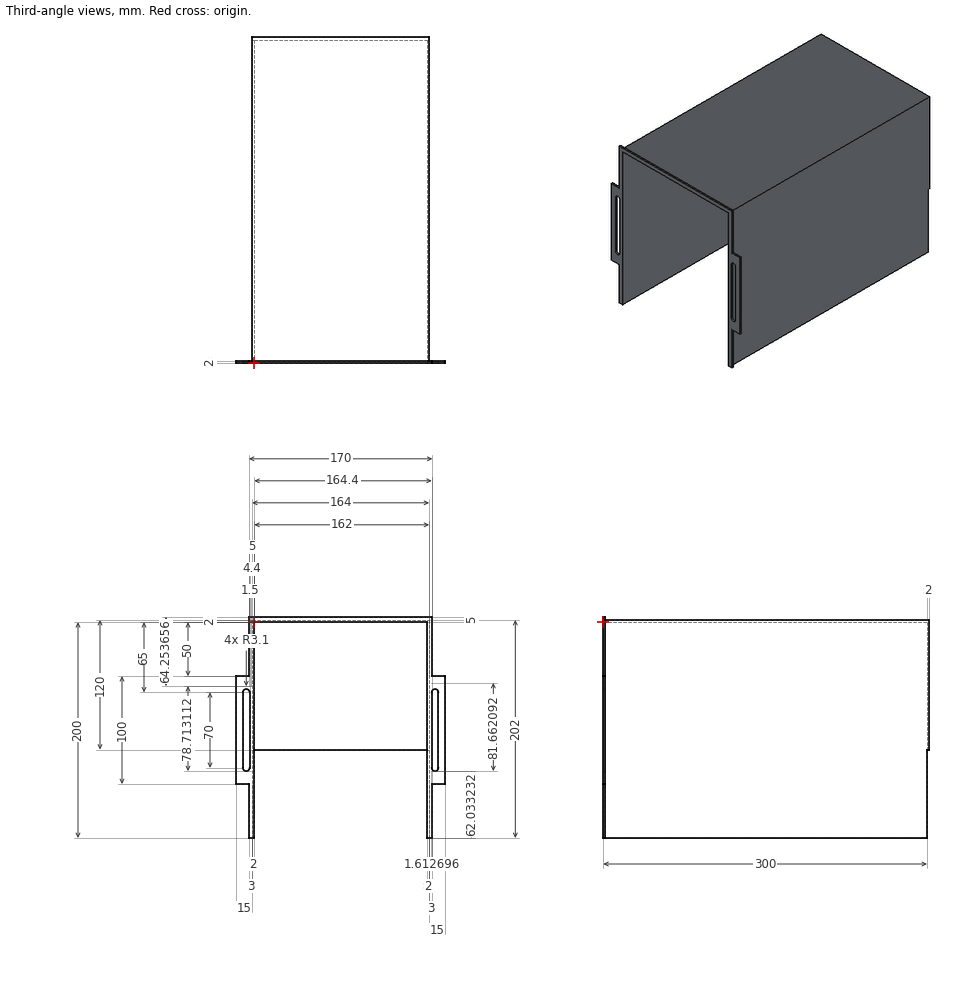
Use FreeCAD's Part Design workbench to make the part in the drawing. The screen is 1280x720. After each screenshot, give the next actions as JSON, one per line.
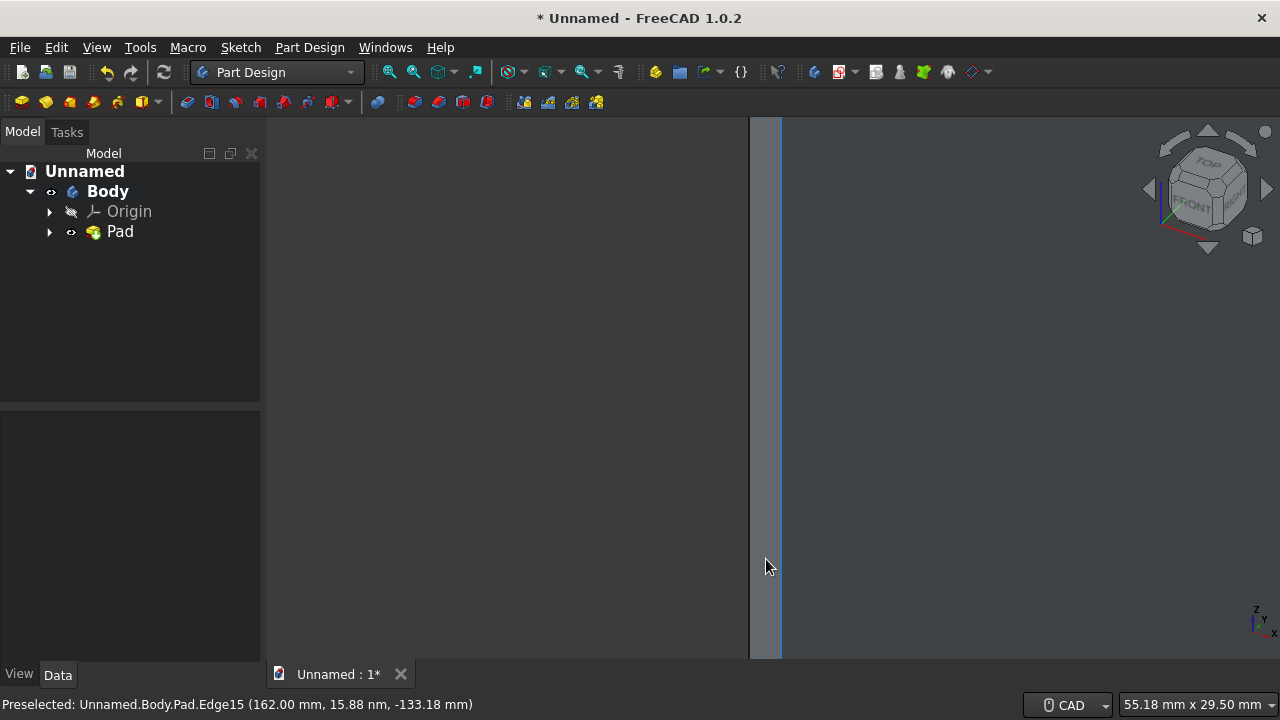
{"action": "left_click", "coordinate": [760, 557]}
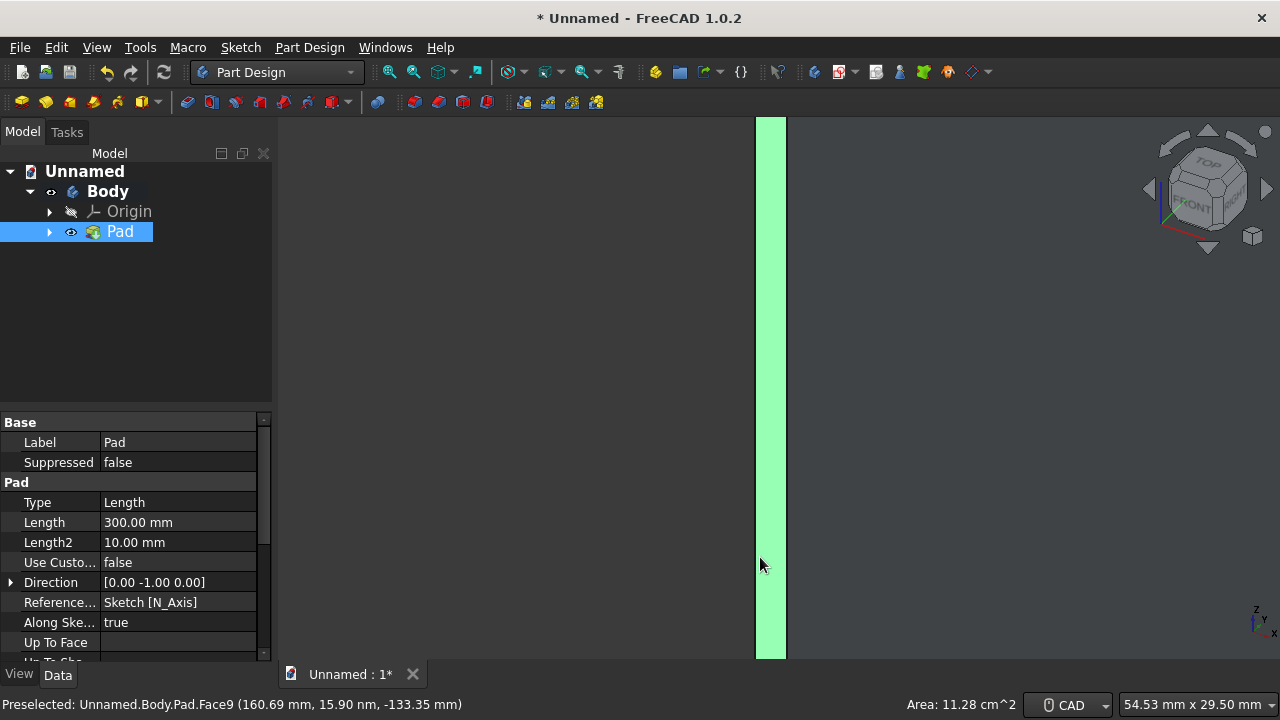
{"action": "left_click", "coordinate": [840, 72]}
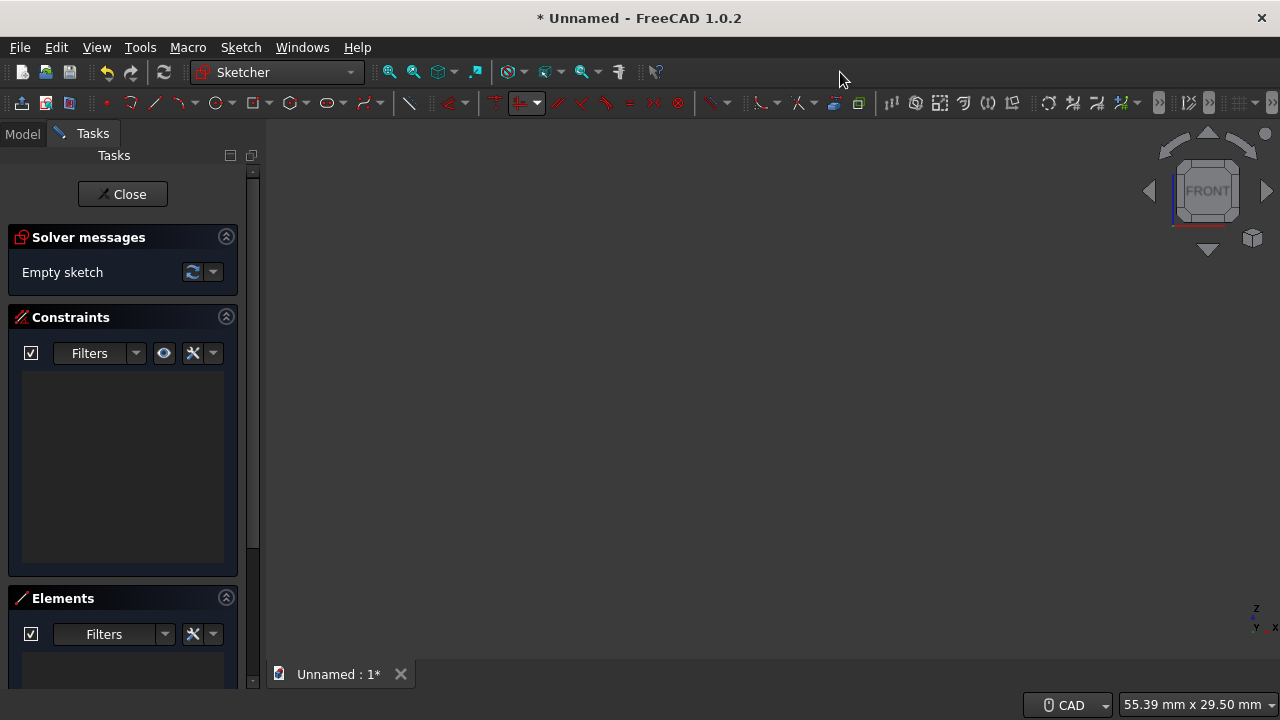
{"action": "scroll", "coordinate": [763, 631], "scroll_direction": "down", "scroll_amount": 11}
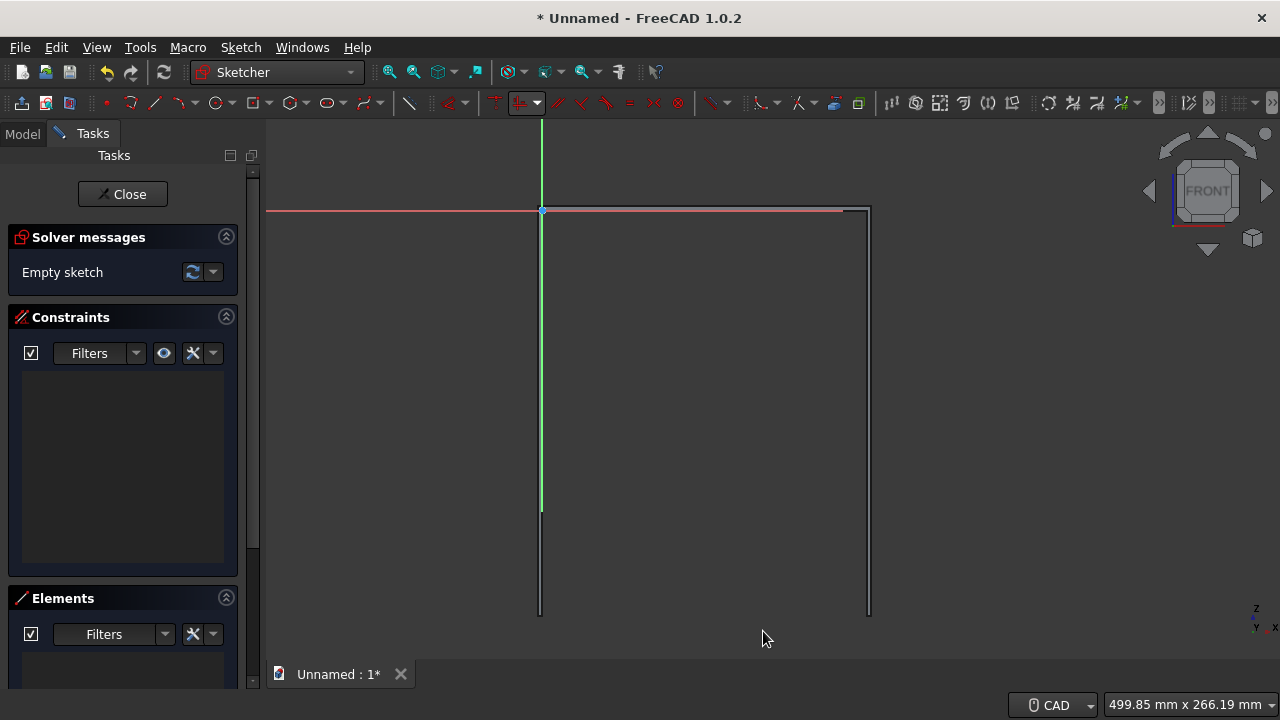
{"action": "left_click", "coordinate": [272, 104]}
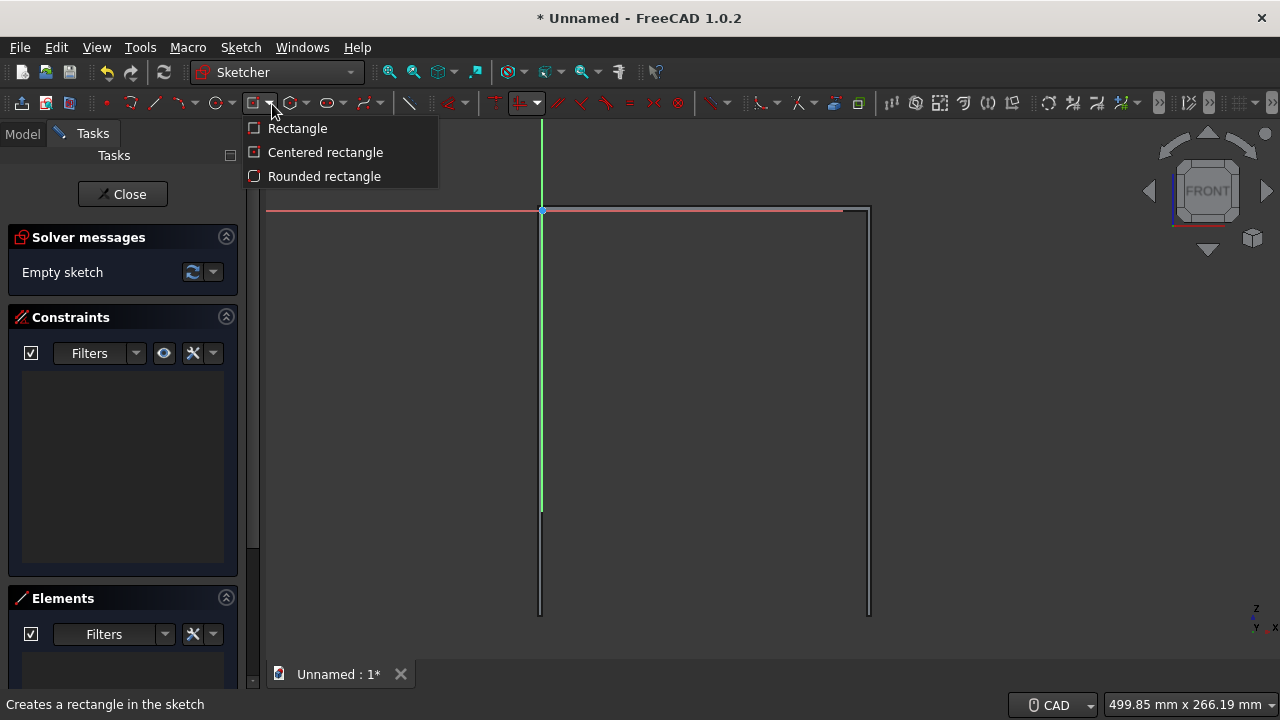
{"action": "left_click", "coordinate": [340, 128]}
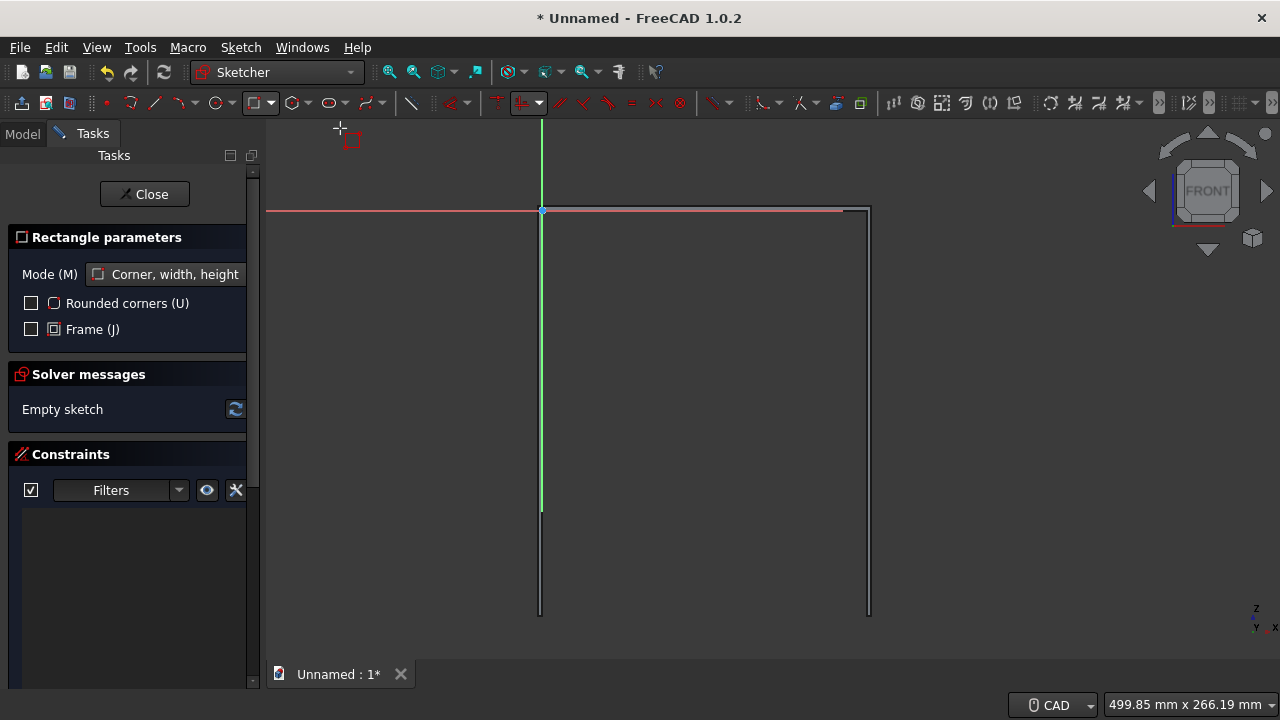
{"action": "left_click", "coordinate": [508, 312]}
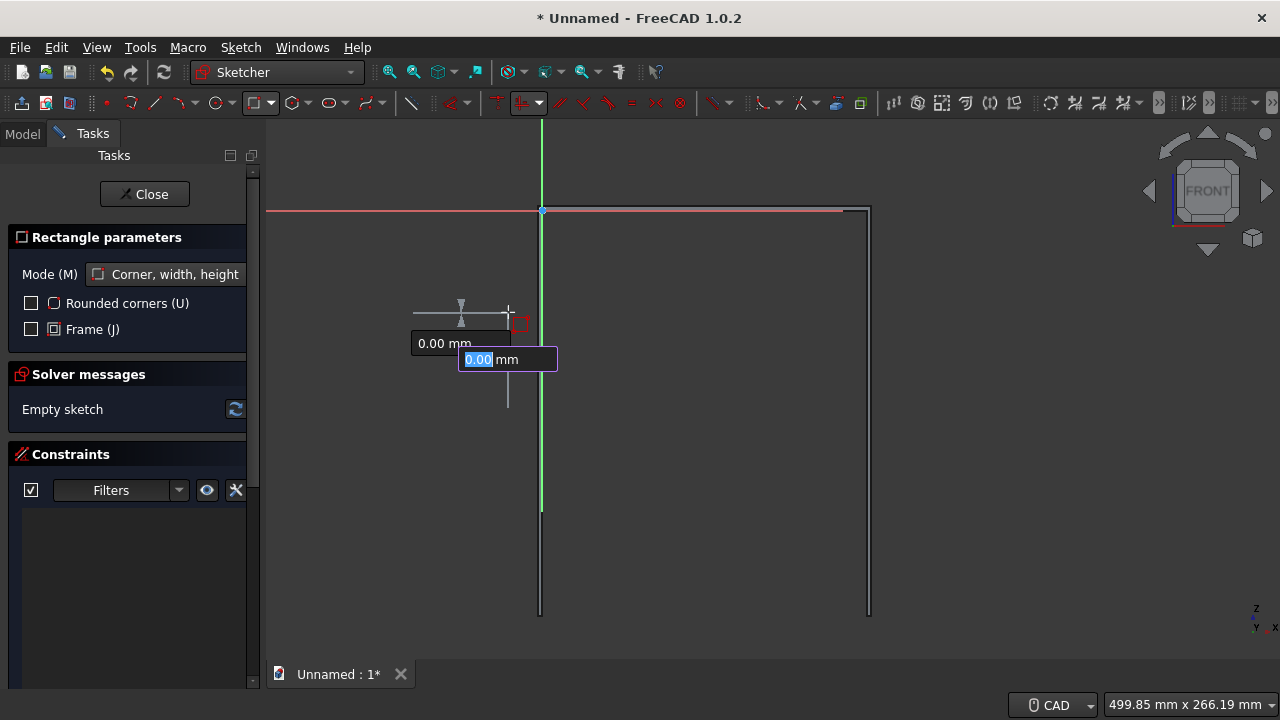
{"action": "scroll", "coordinate": [538, 515], "scroll_direction": "up", "scroll_amount": 7}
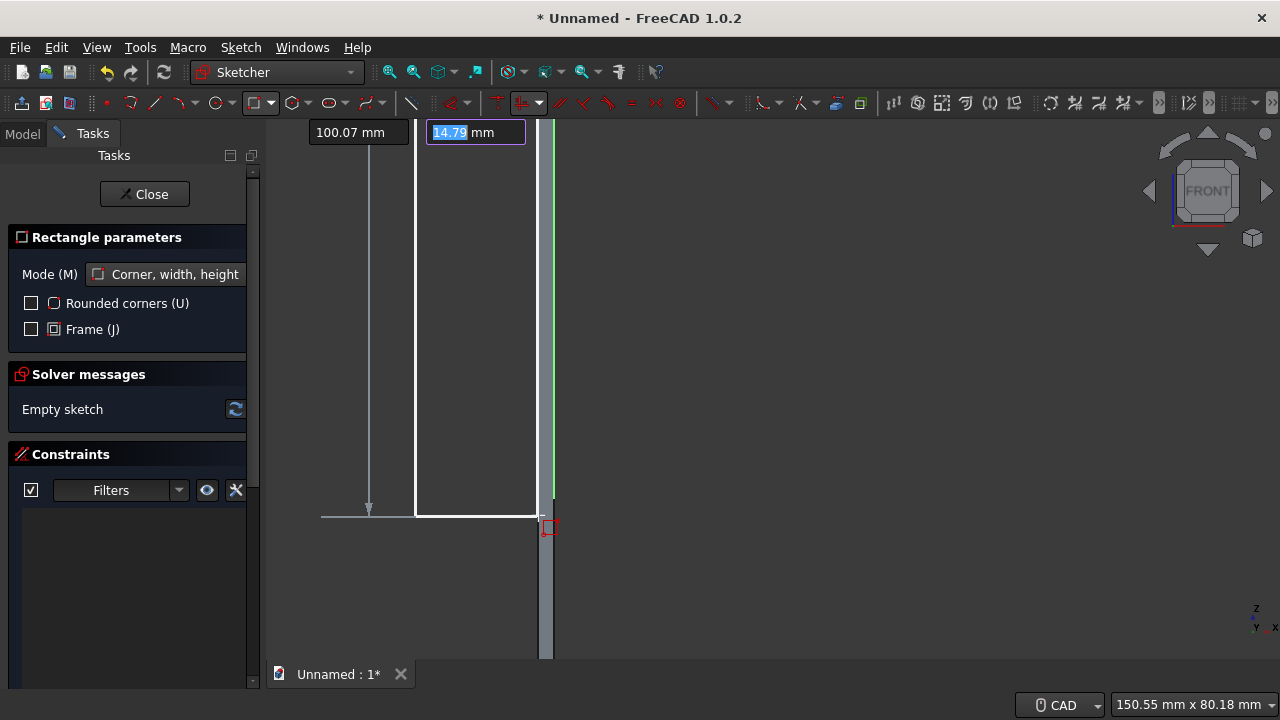
{"action": "left_click", "coordinate": [538, 512]}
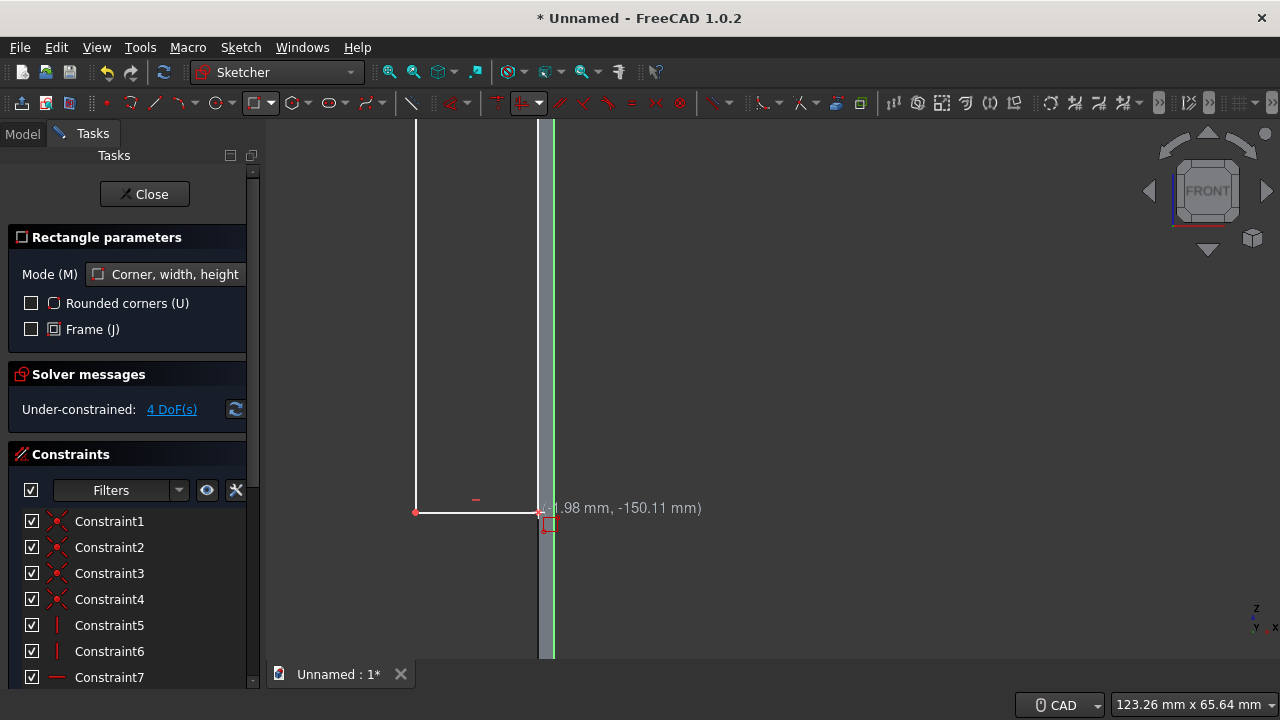
{"action": "scroll", "coordinate": [486, 602], "scroll_direction": "down", "scroll_amount": 6}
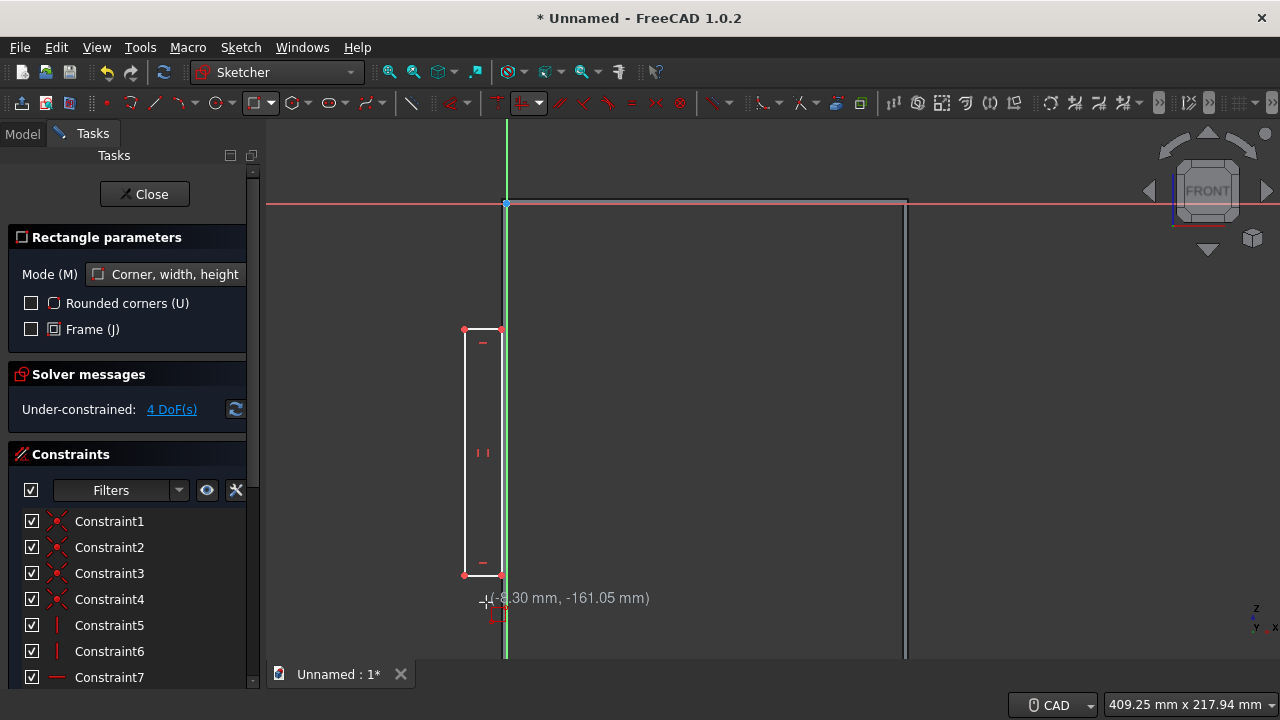
{"action": "left_click", "coordinate": [908, 328]}
{"action": "left_click", "coordinate": [945, 576]}
{"action": "key", "text": "Escape"}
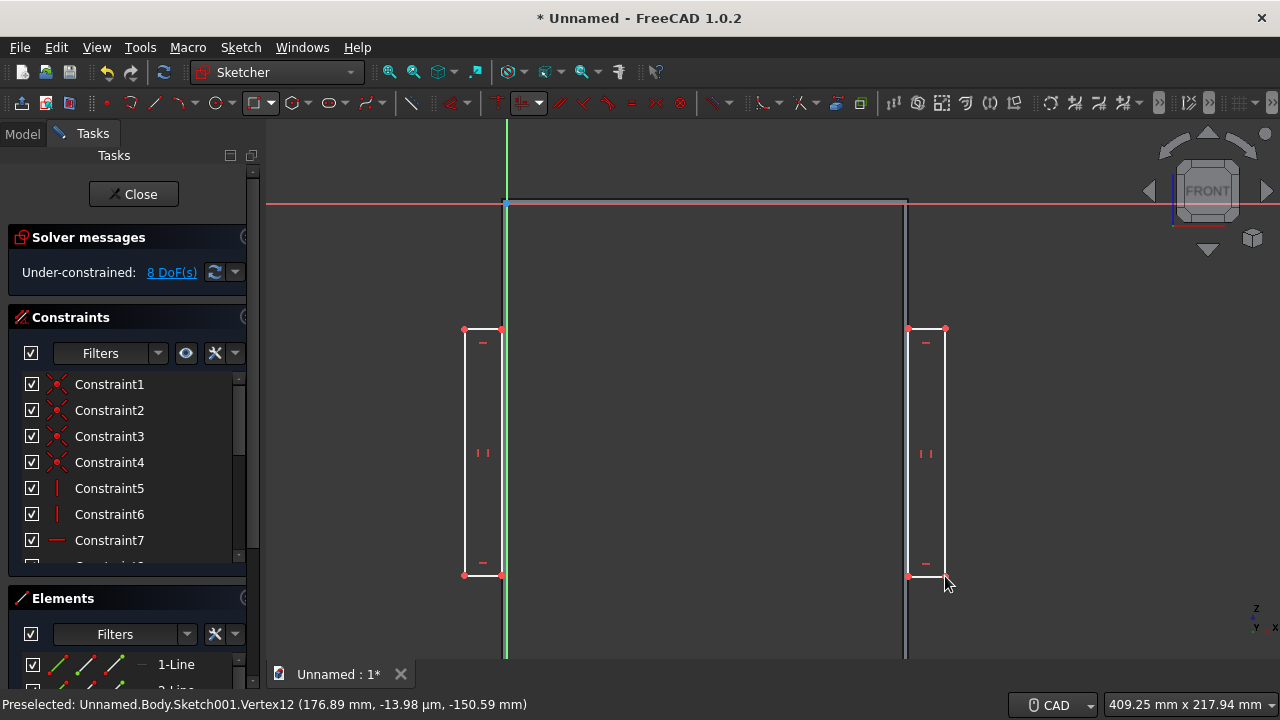
{"action": "left_click", "coordinate": [450, 104]}